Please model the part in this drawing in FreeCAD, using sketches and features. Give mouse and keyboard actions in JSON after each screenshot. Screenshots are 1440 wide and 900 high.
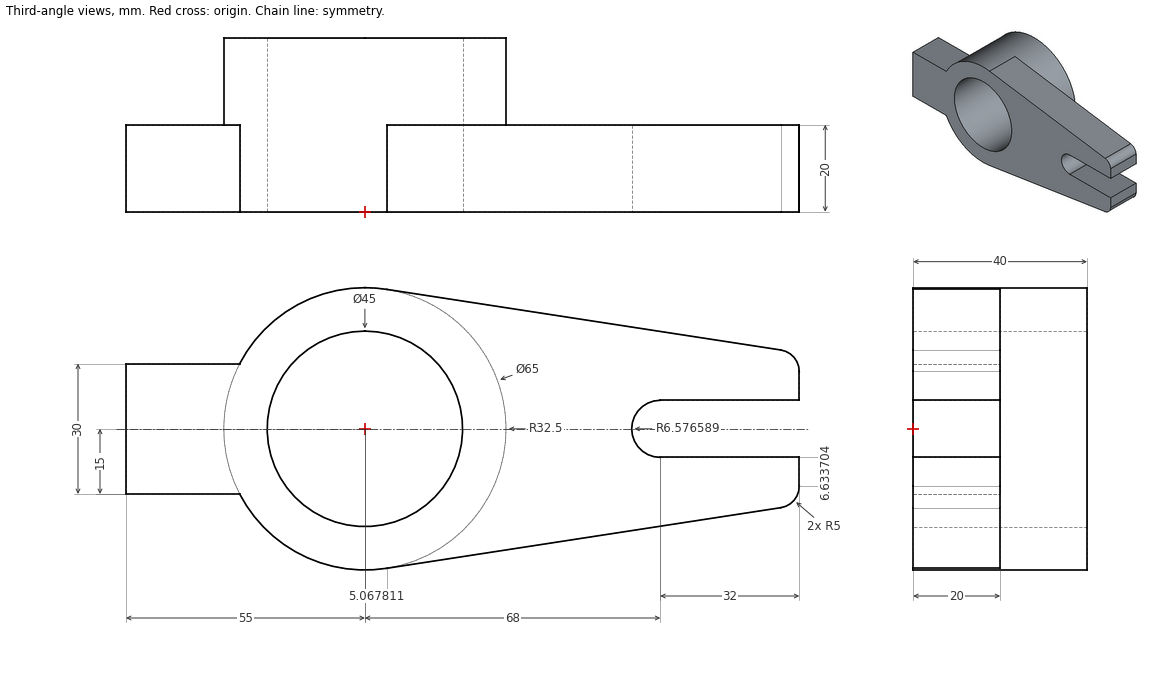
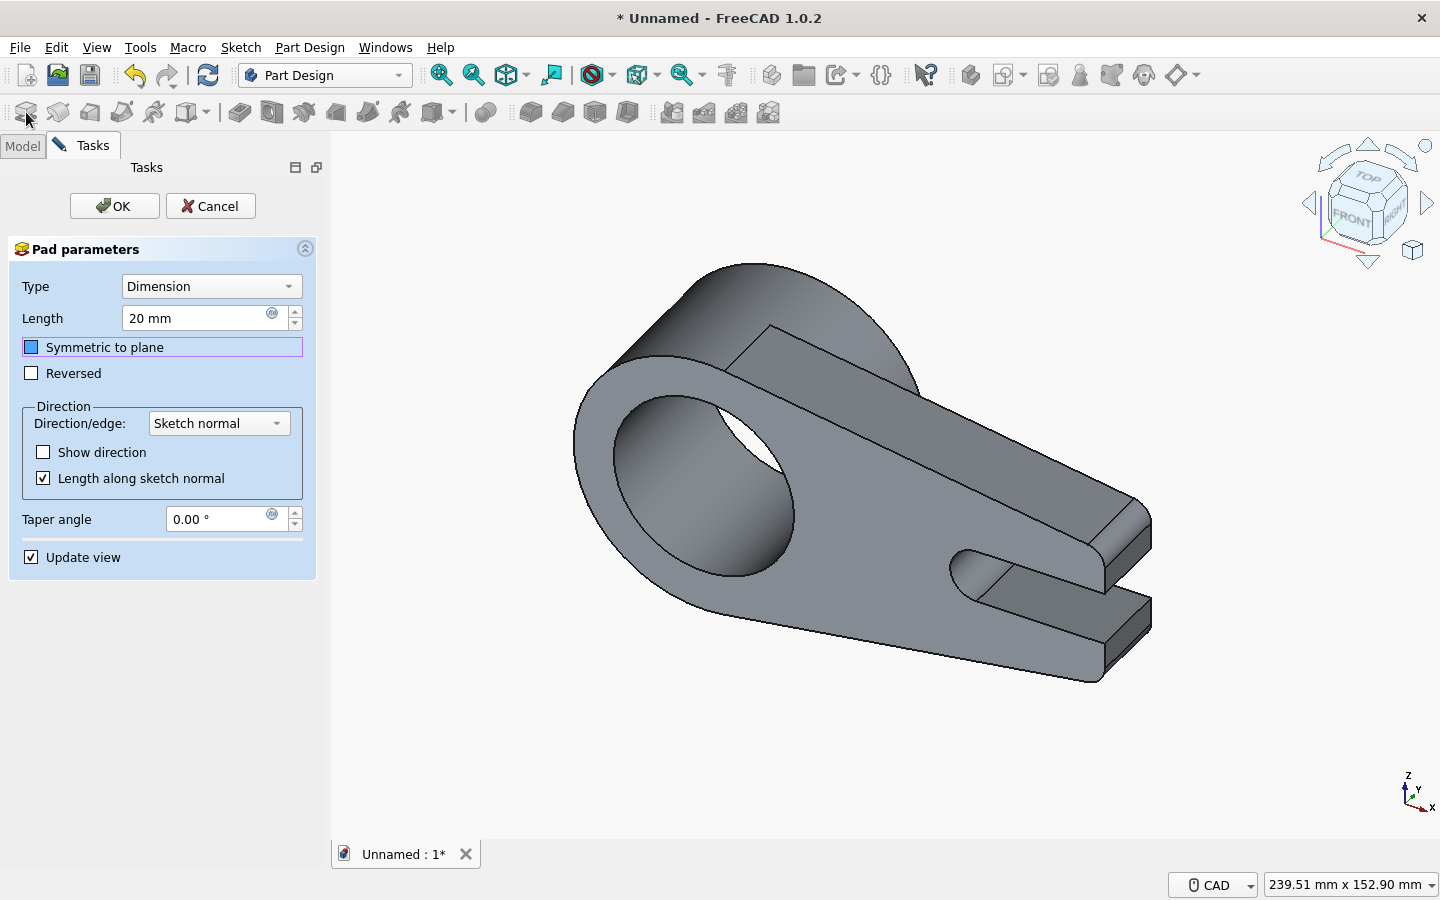
{"action": "left_click", "coordinate": [30, 373]}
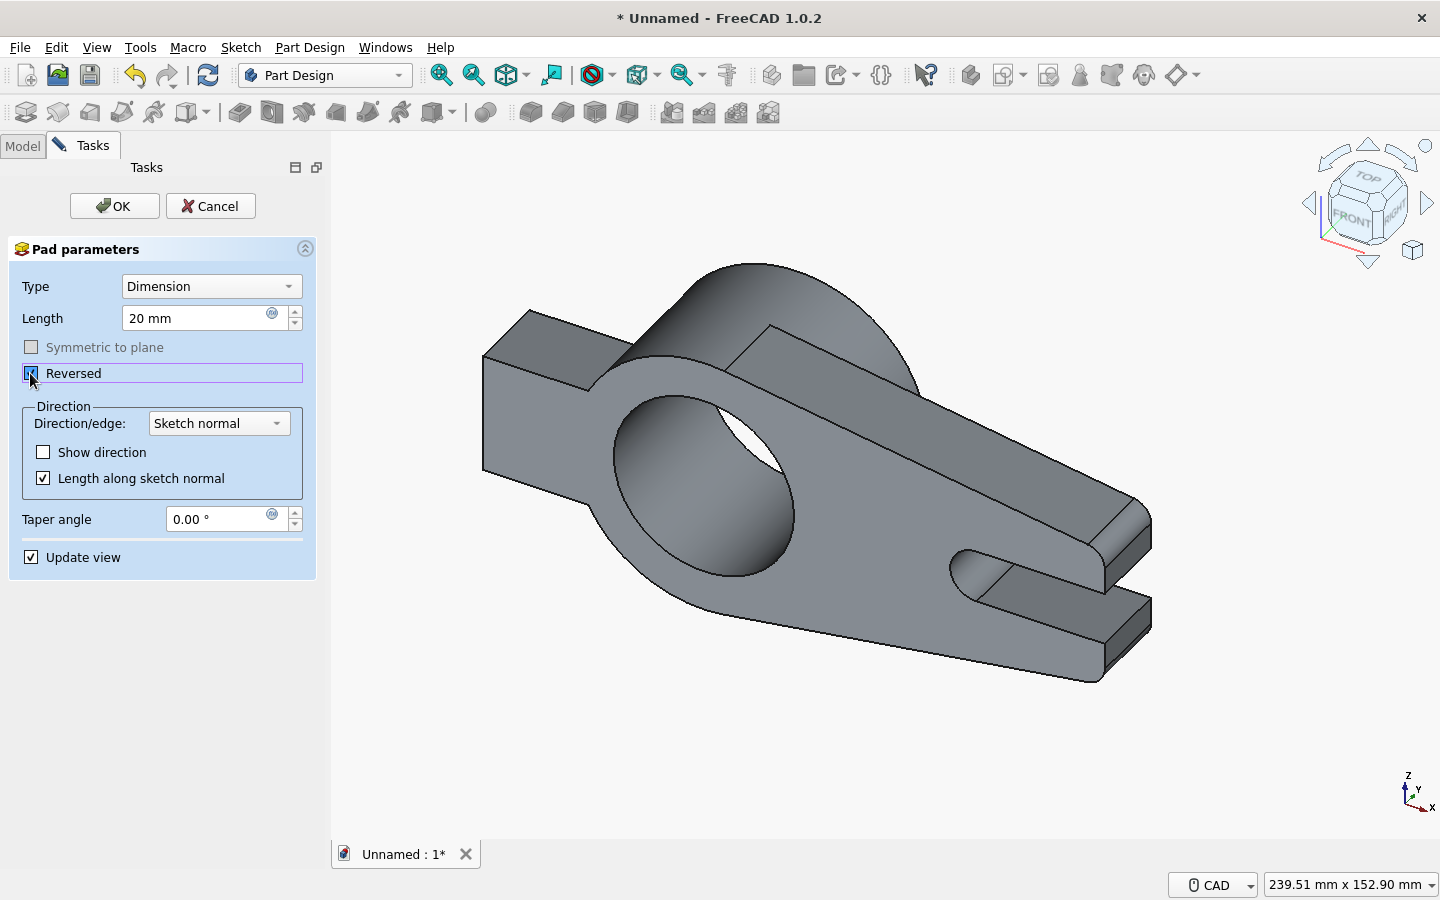
{"action": "left_click", "coordinate": [115, 206]}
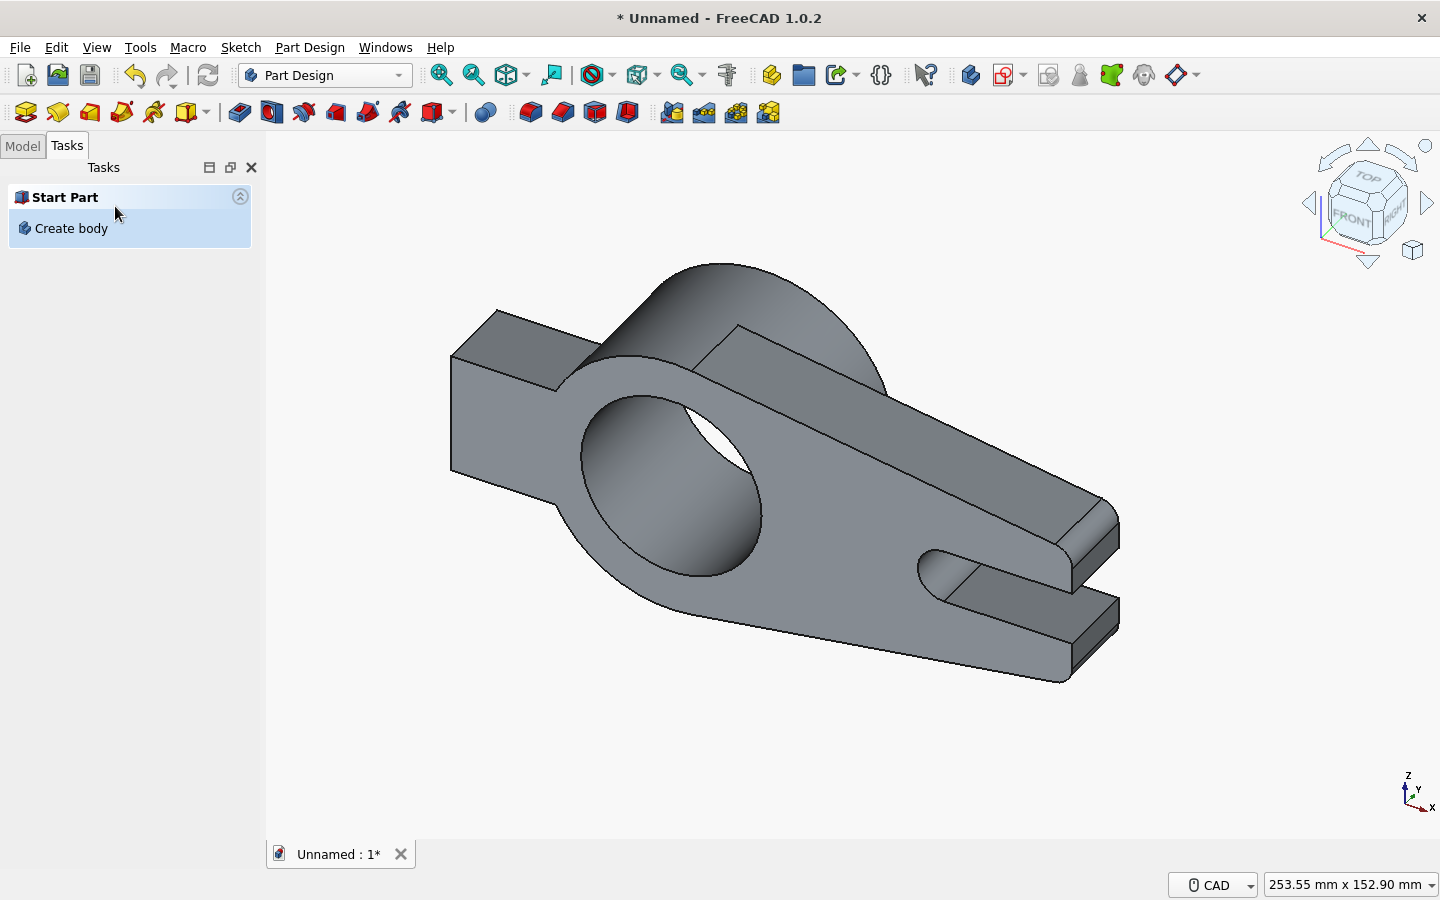
{"action": "key", "text": "0"}